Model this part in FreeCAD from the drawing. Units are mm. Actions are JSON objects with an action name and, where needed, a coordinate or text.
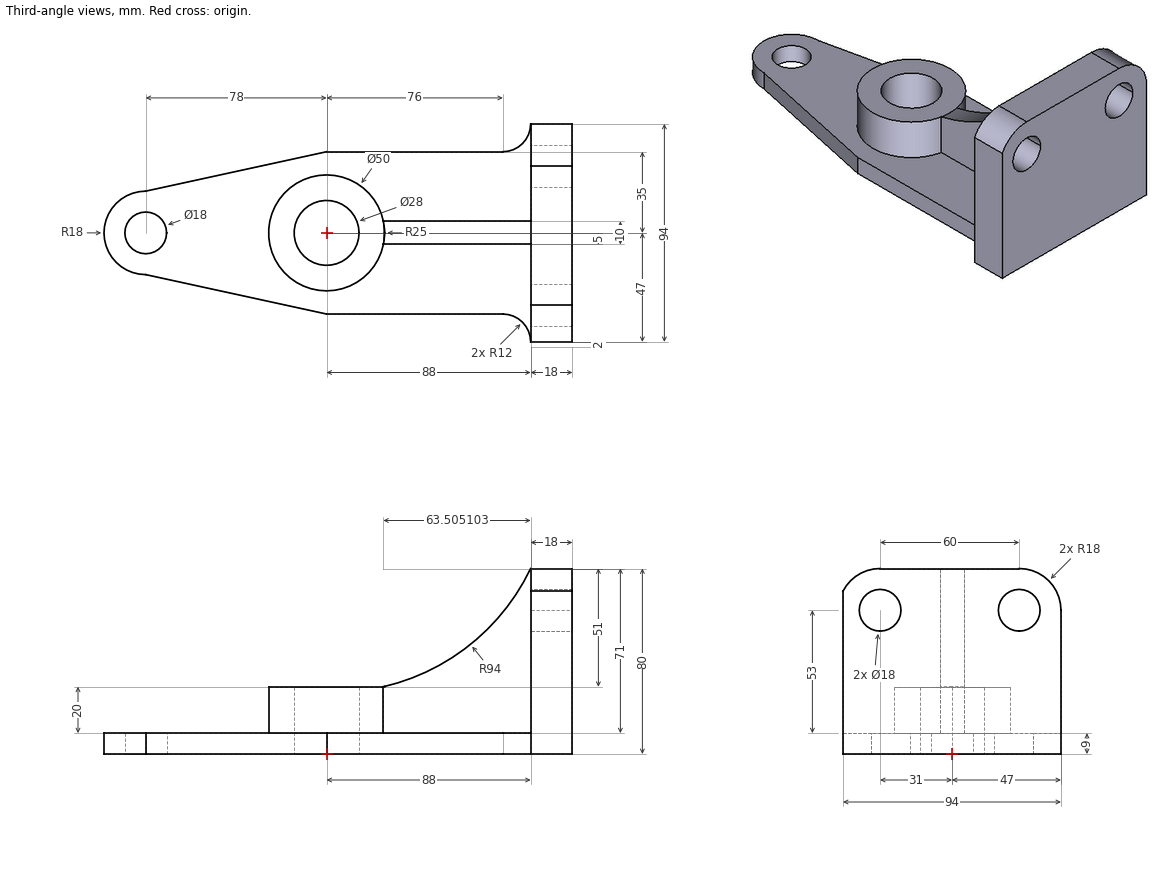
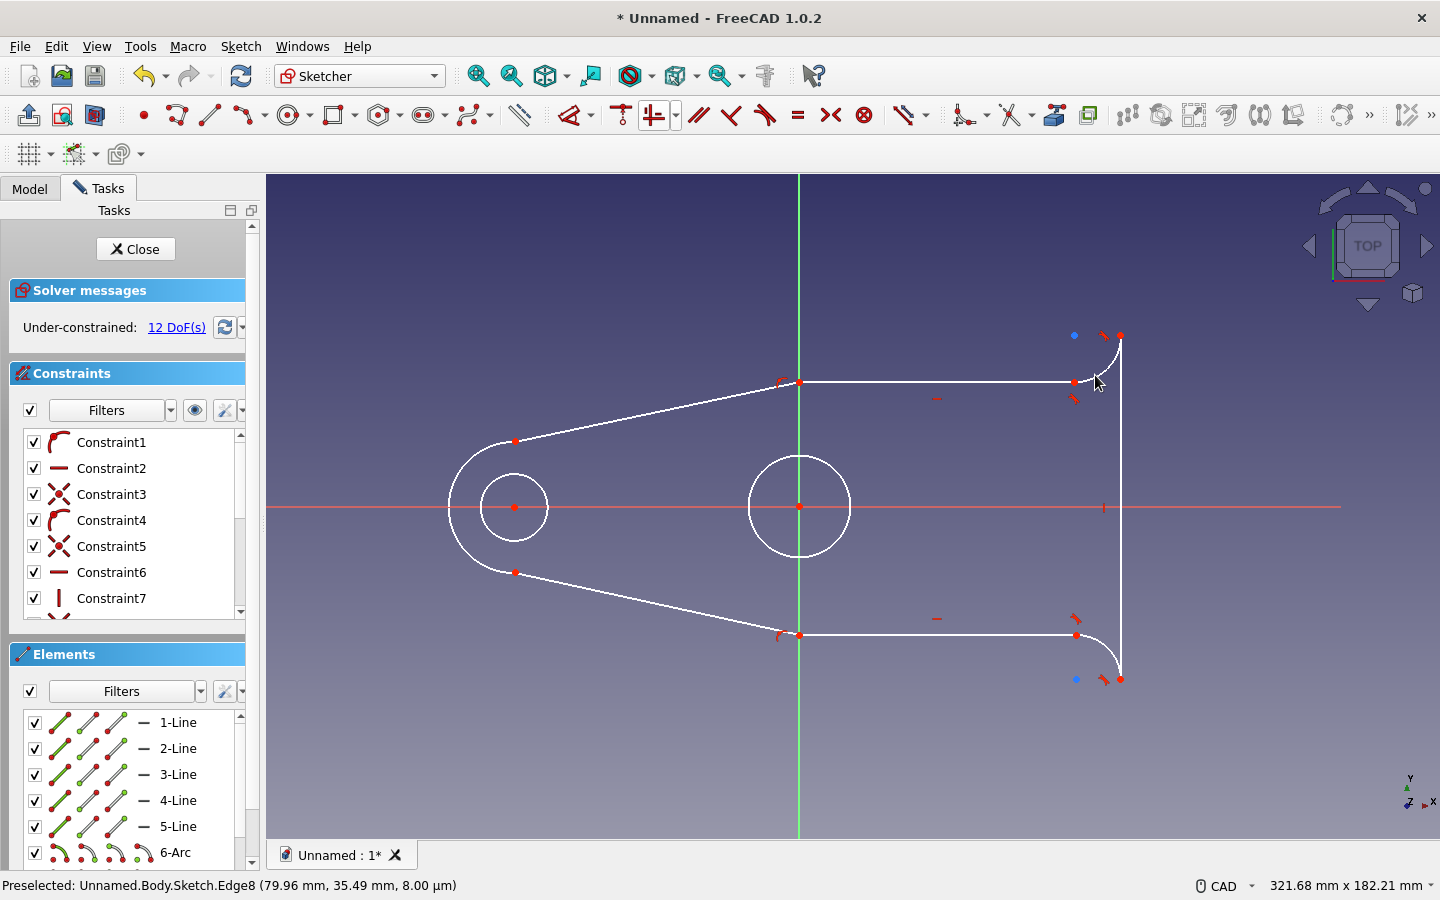
{"action": "left_click", "coordinate": [1096, 640]}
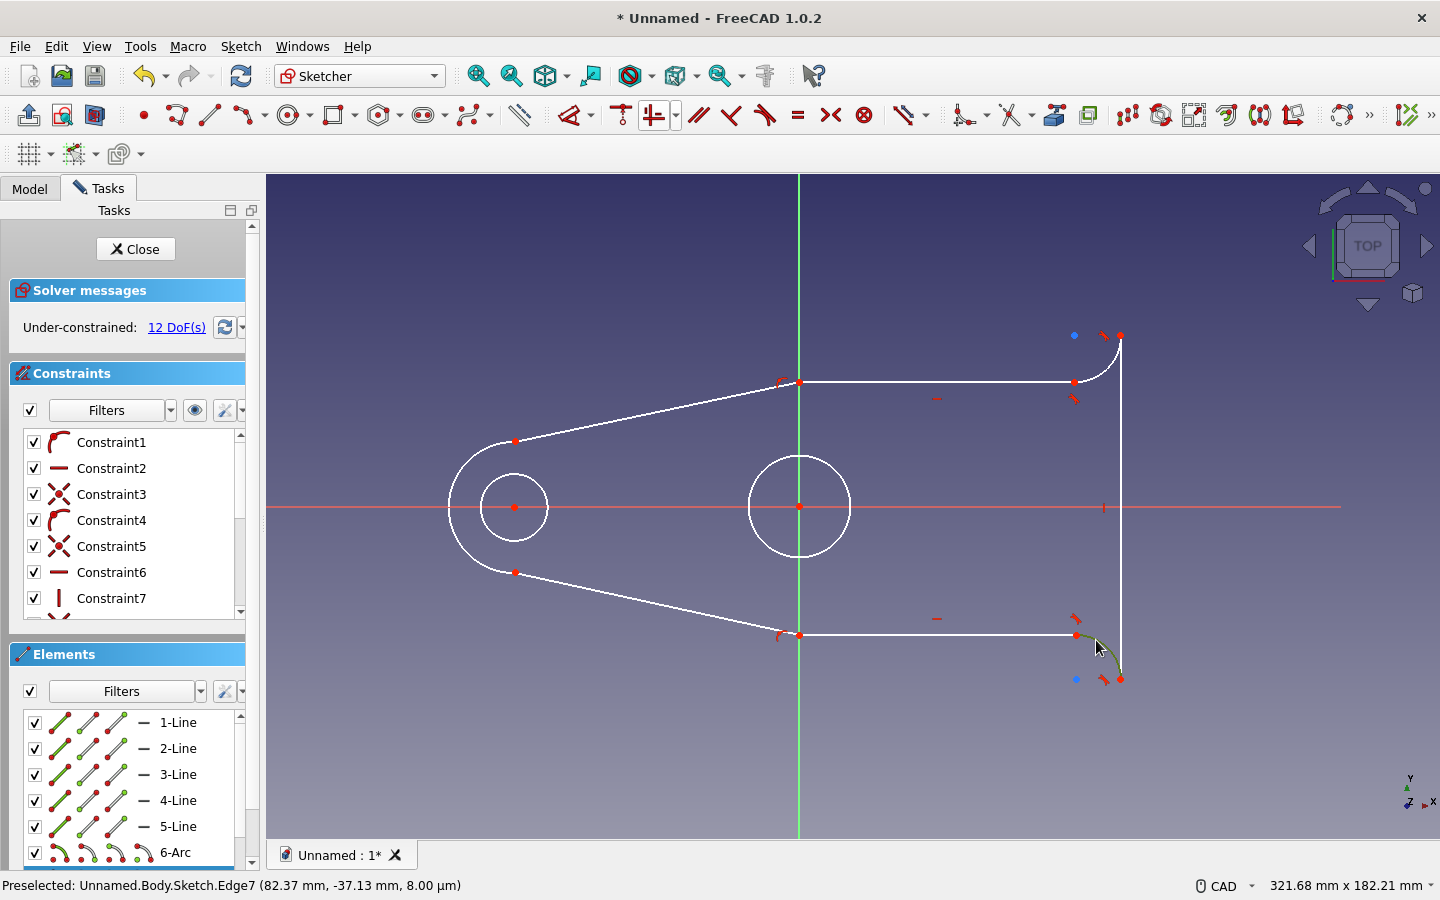
{"action": "left_click", "coordinate": [1096, 377]}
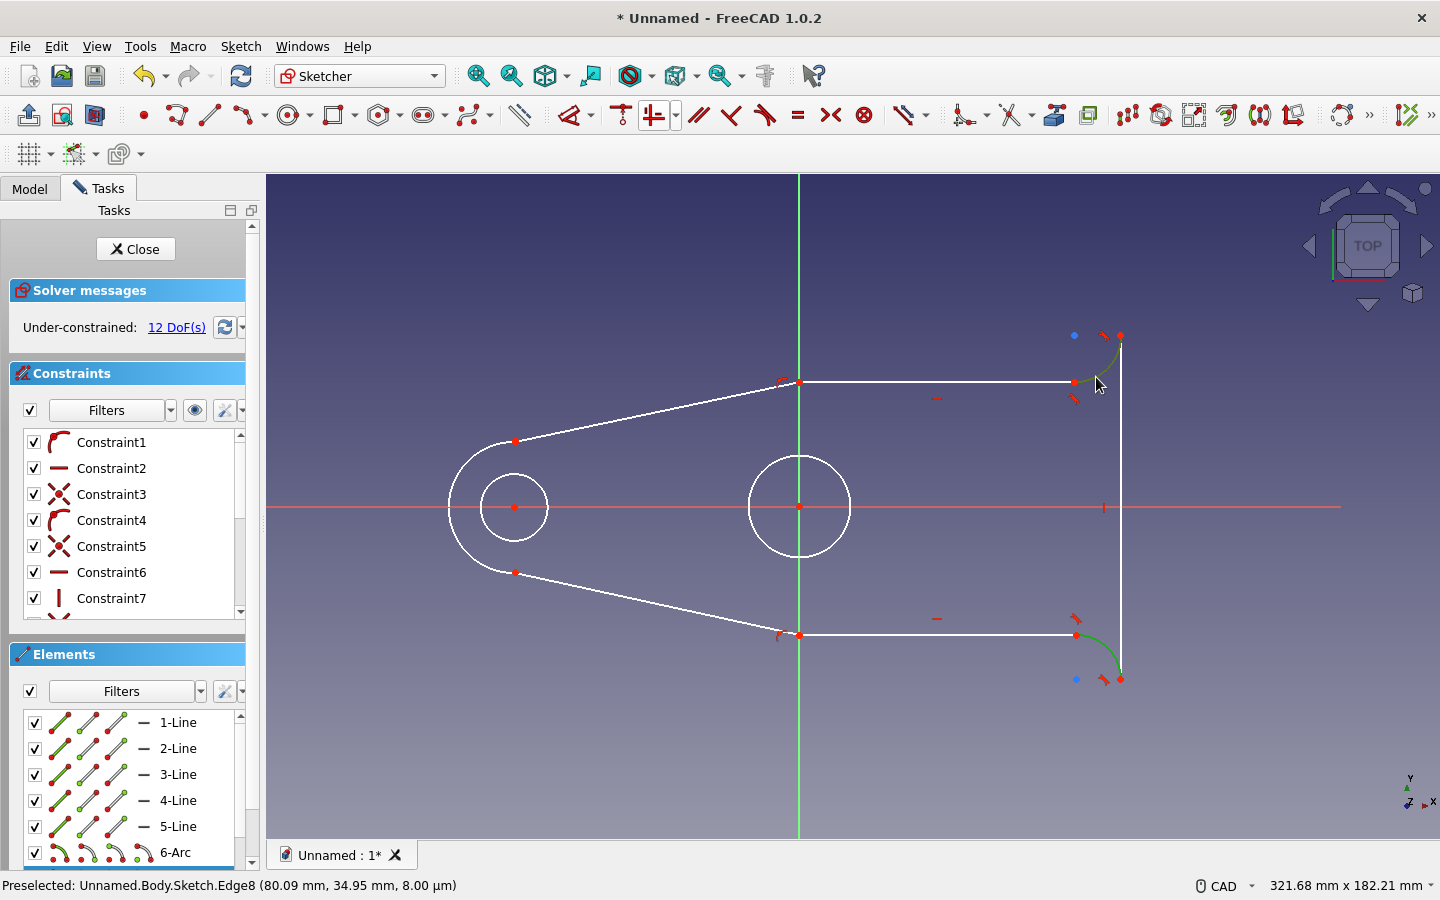
{"action": "left_click", "coordinate": [798, 116]}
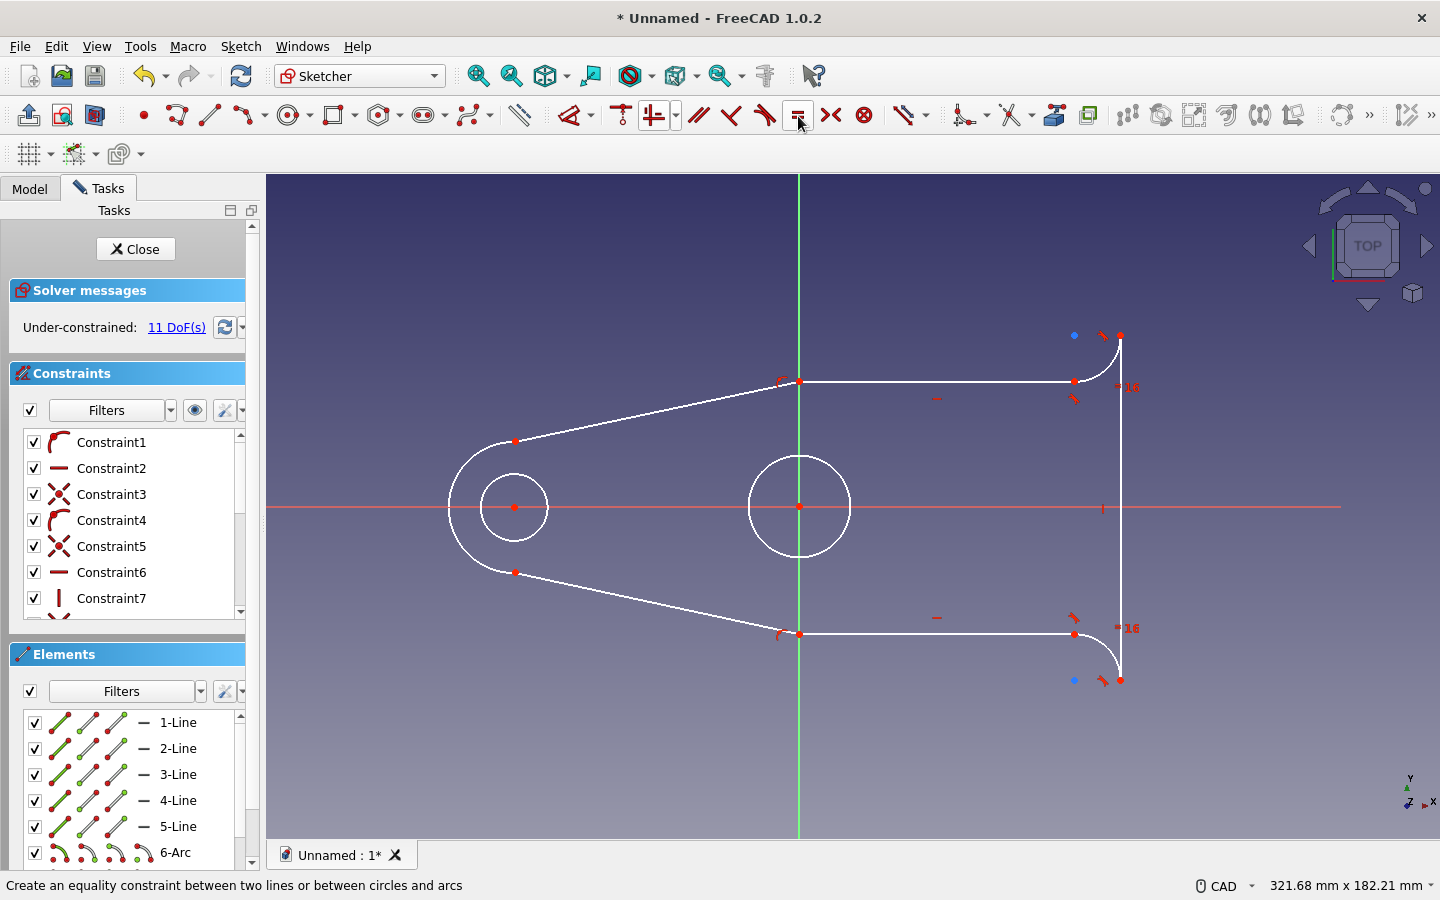
{"action": "left_click", "coordinate": [514, 508]}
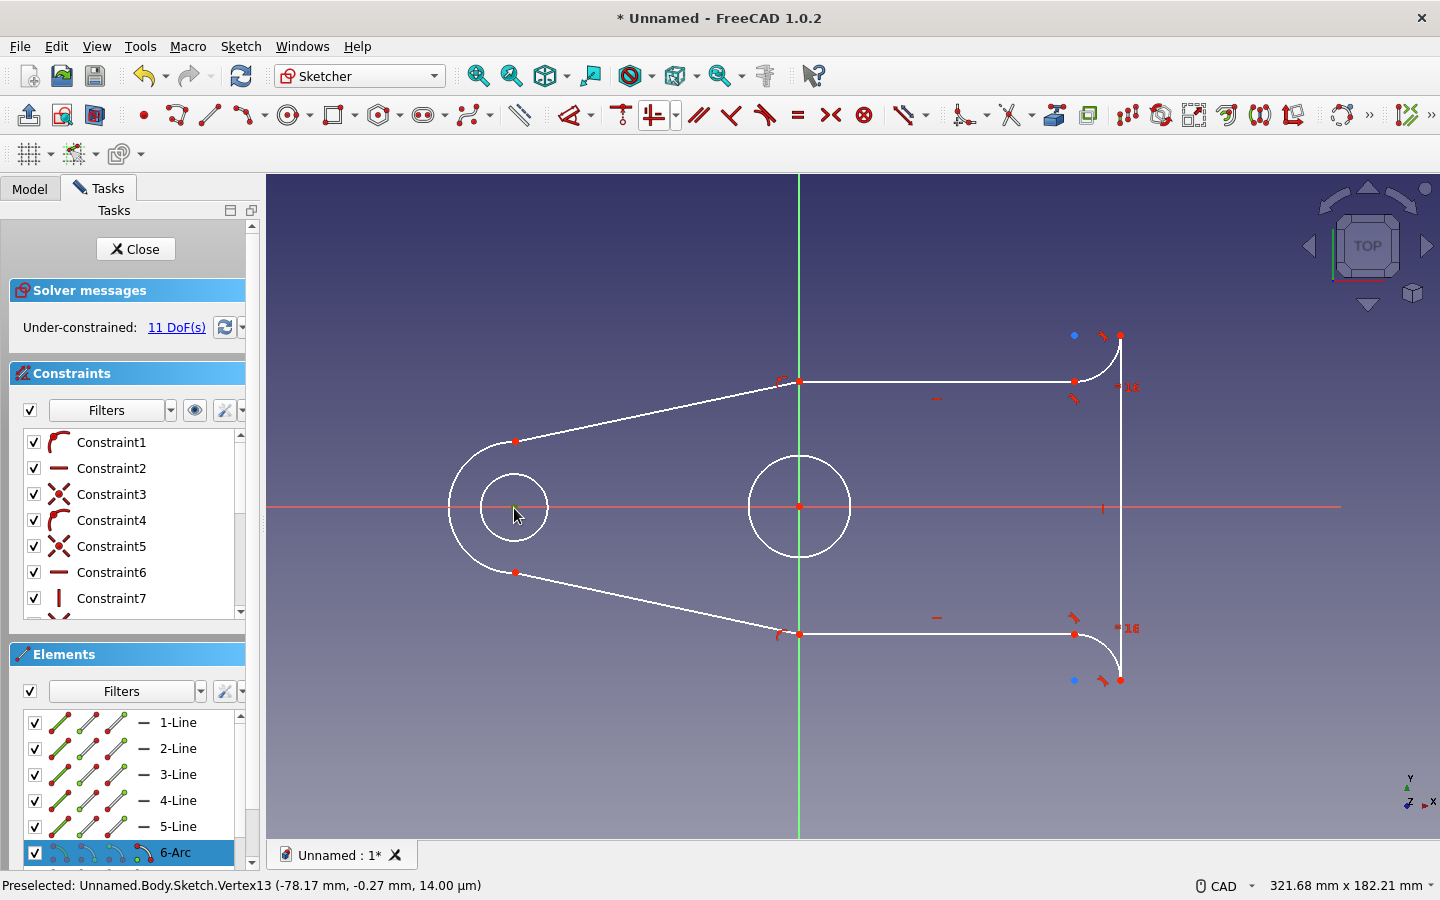
{"action": "left_click", "coordinate": [364, 507]}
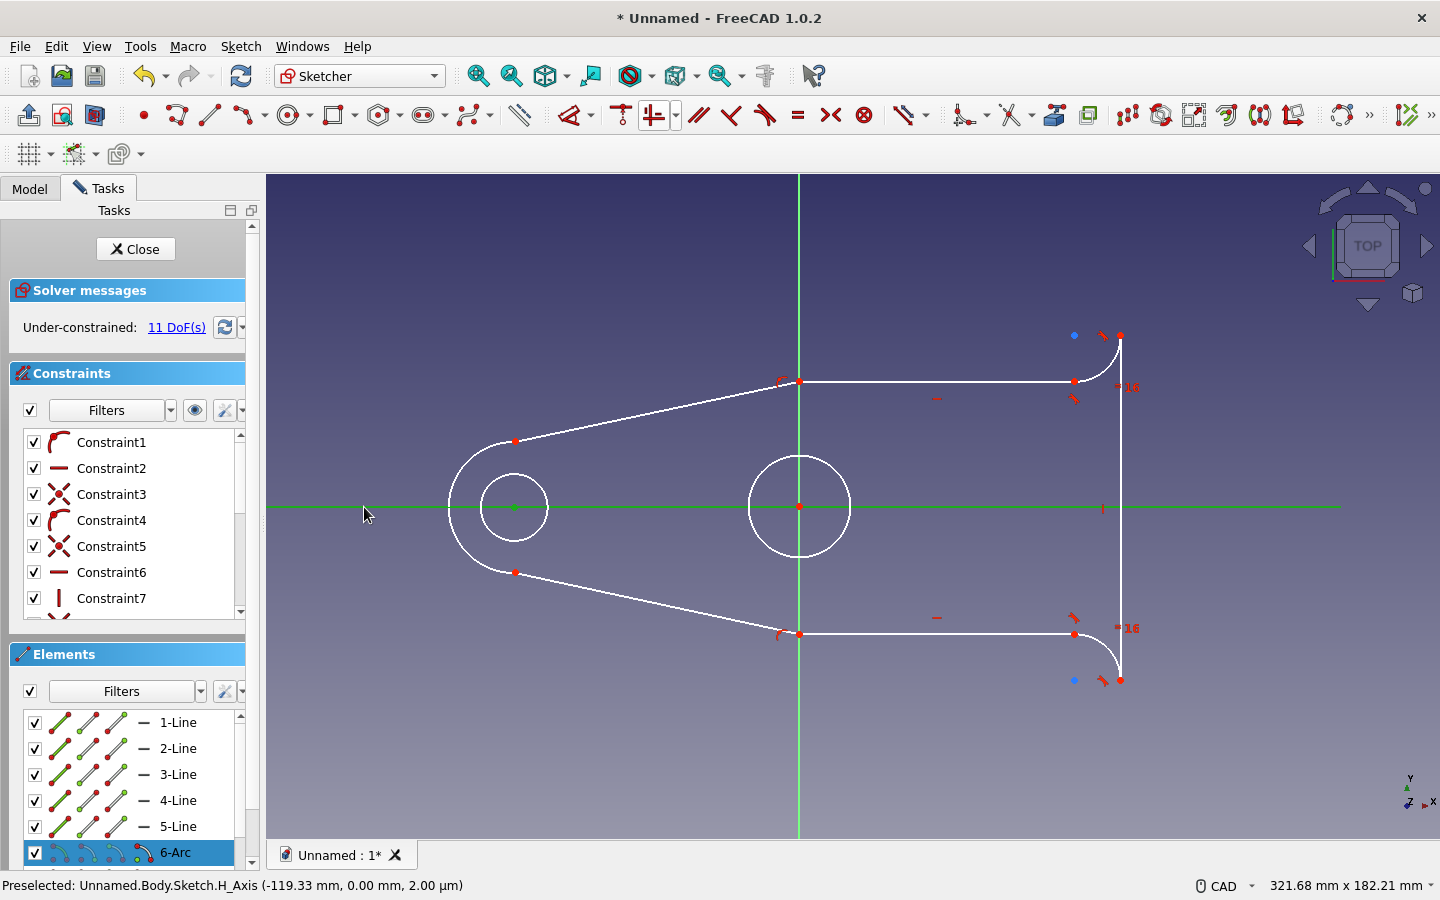
{"action": "left_click", "coordinate": [621, 116]}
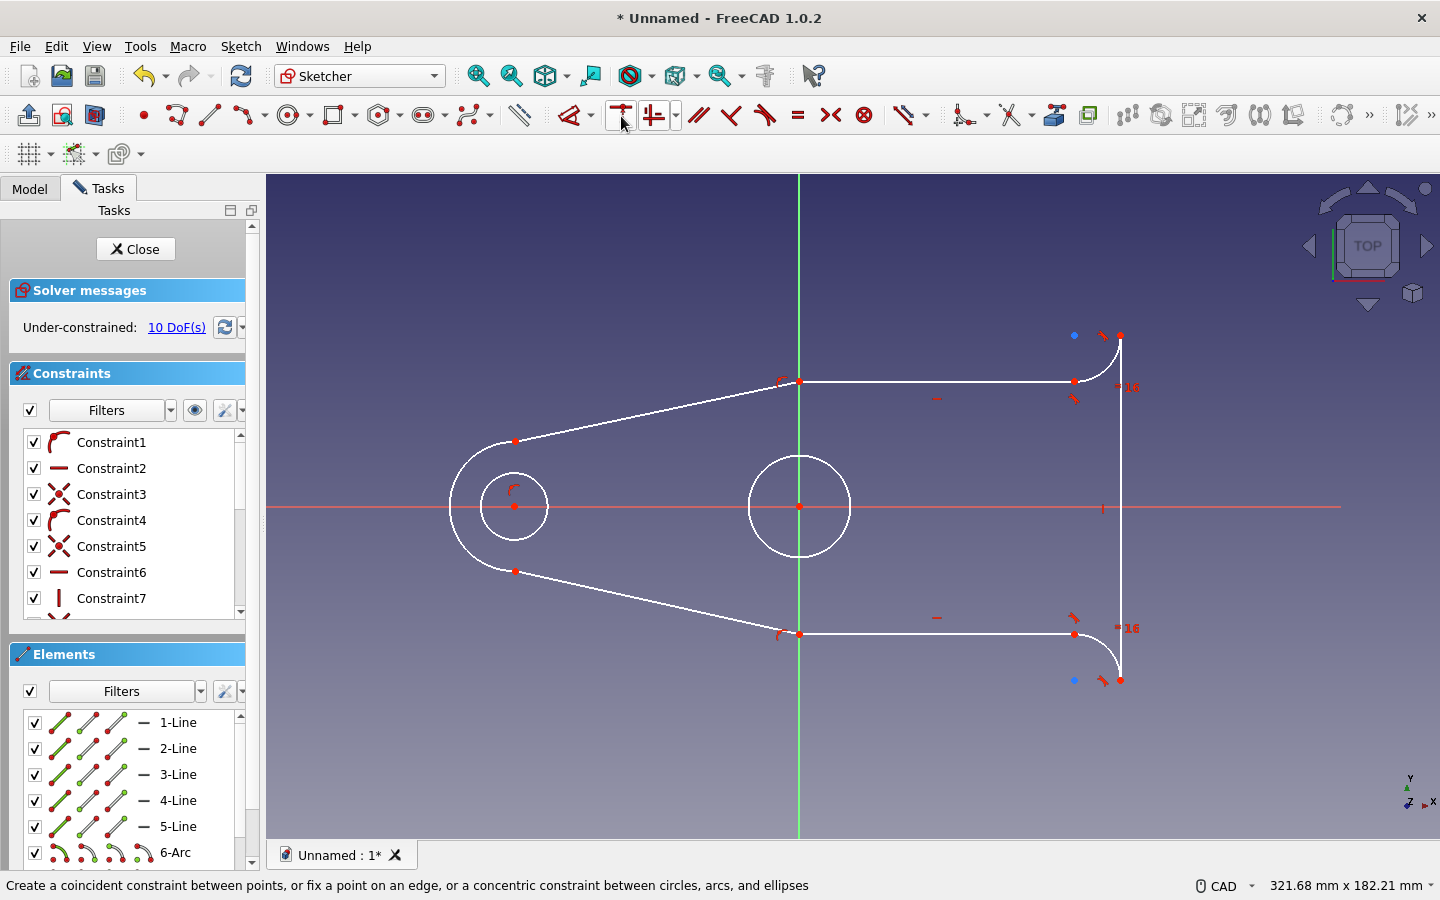
{"action": "left_click", "coordinate": [568, 116]}